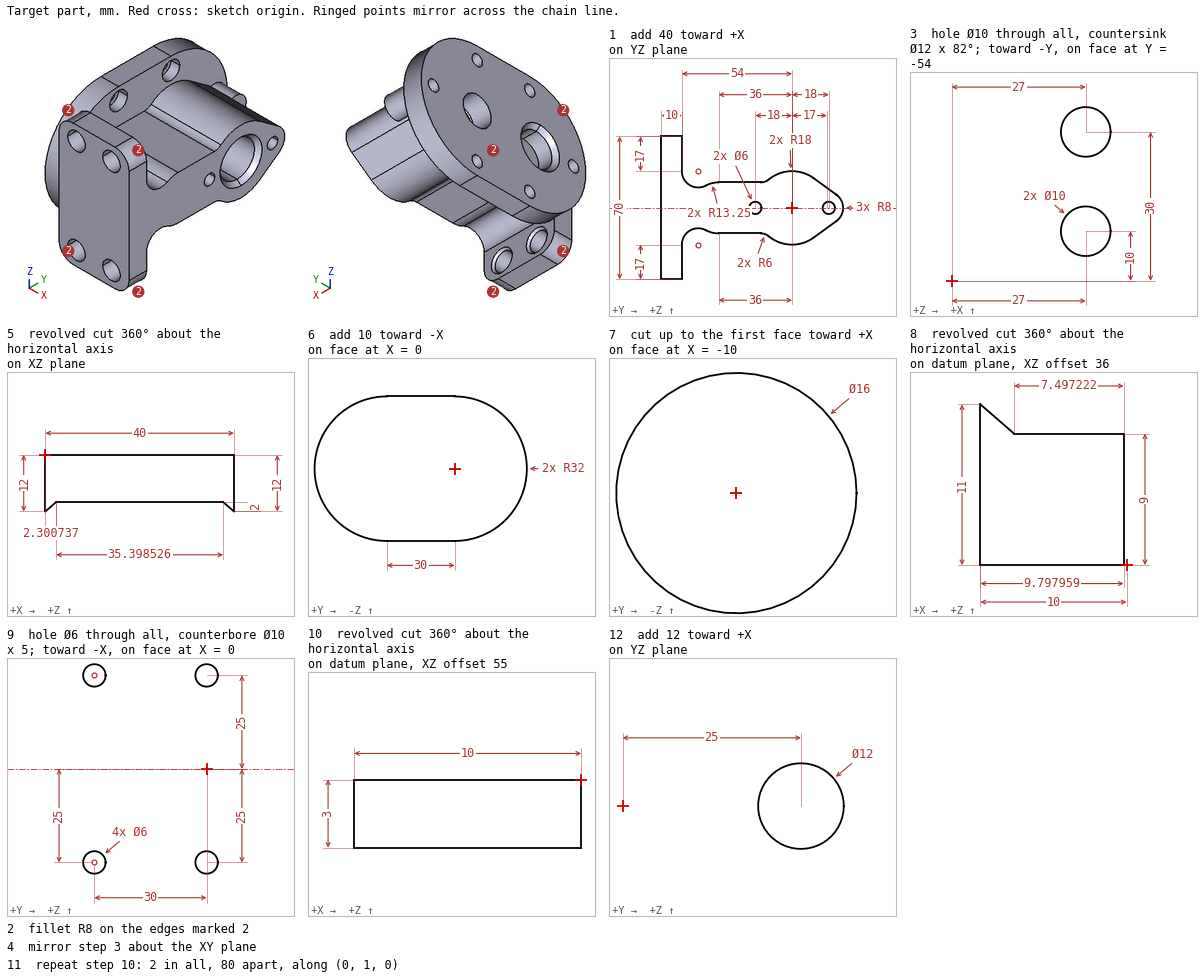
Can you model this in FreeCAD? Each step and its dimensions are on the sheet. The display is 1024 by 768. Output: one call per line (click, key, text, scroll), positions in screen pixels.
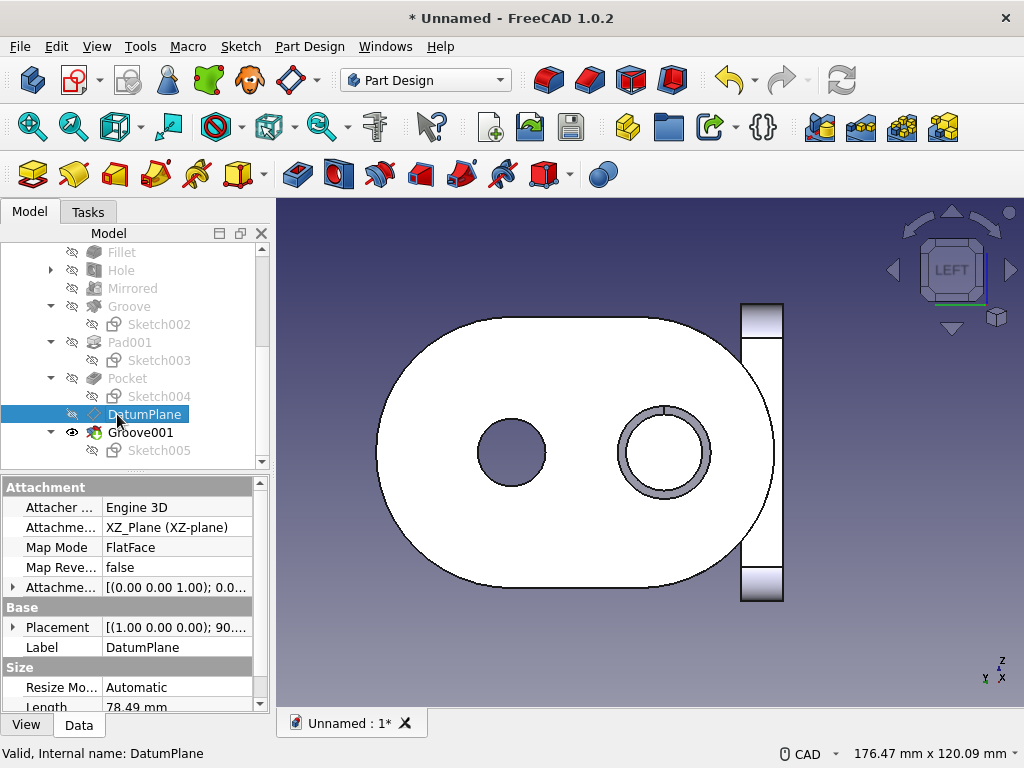
key(0)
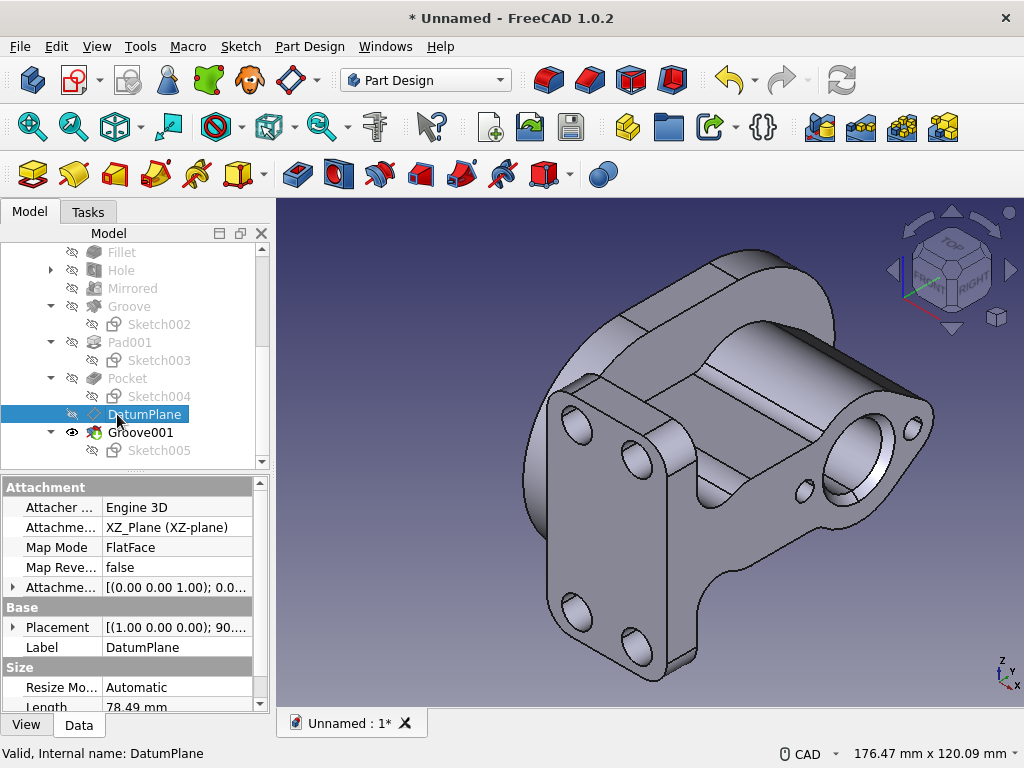
click(33, 128)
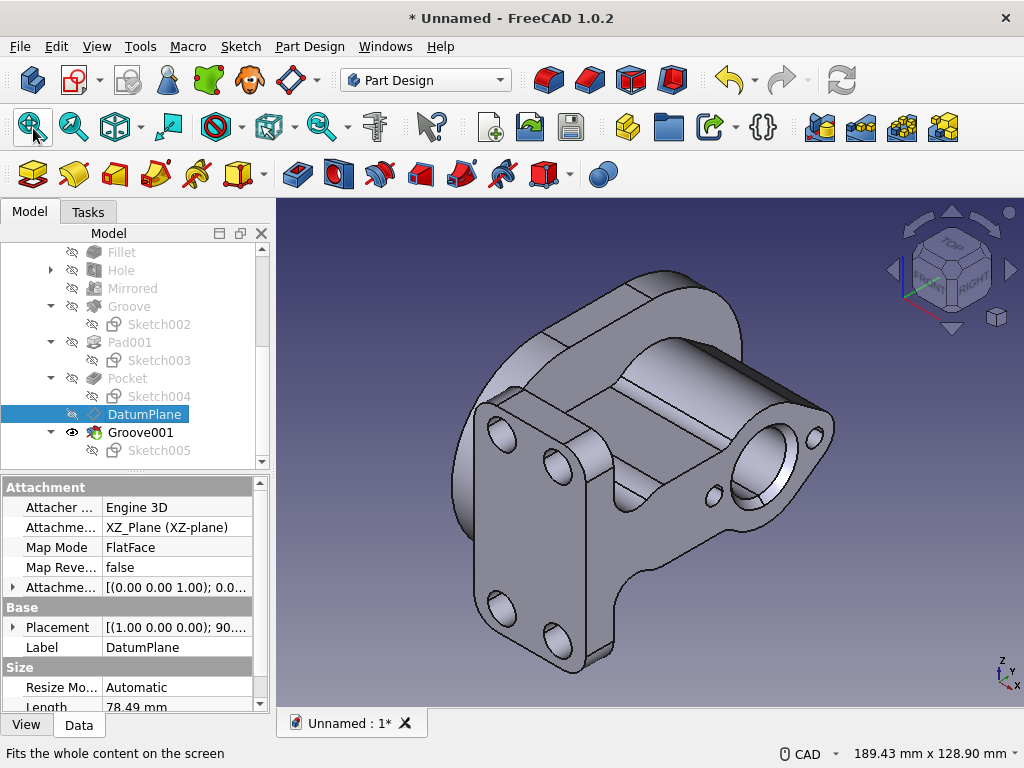
click(588, 380)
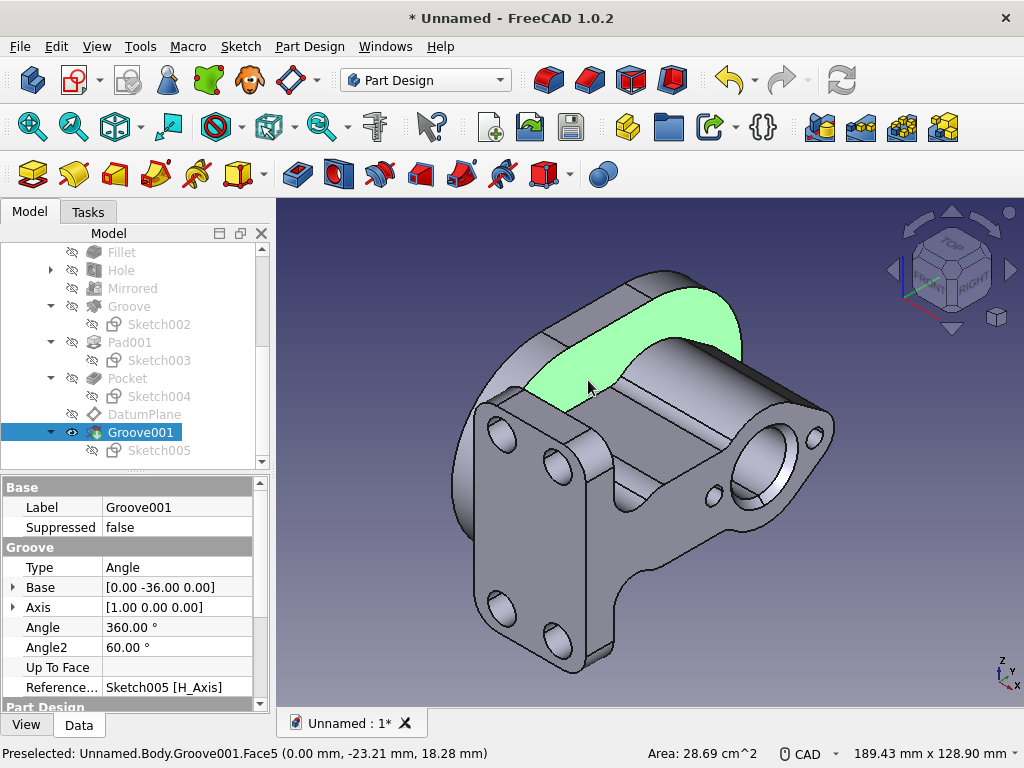
click(74, 80)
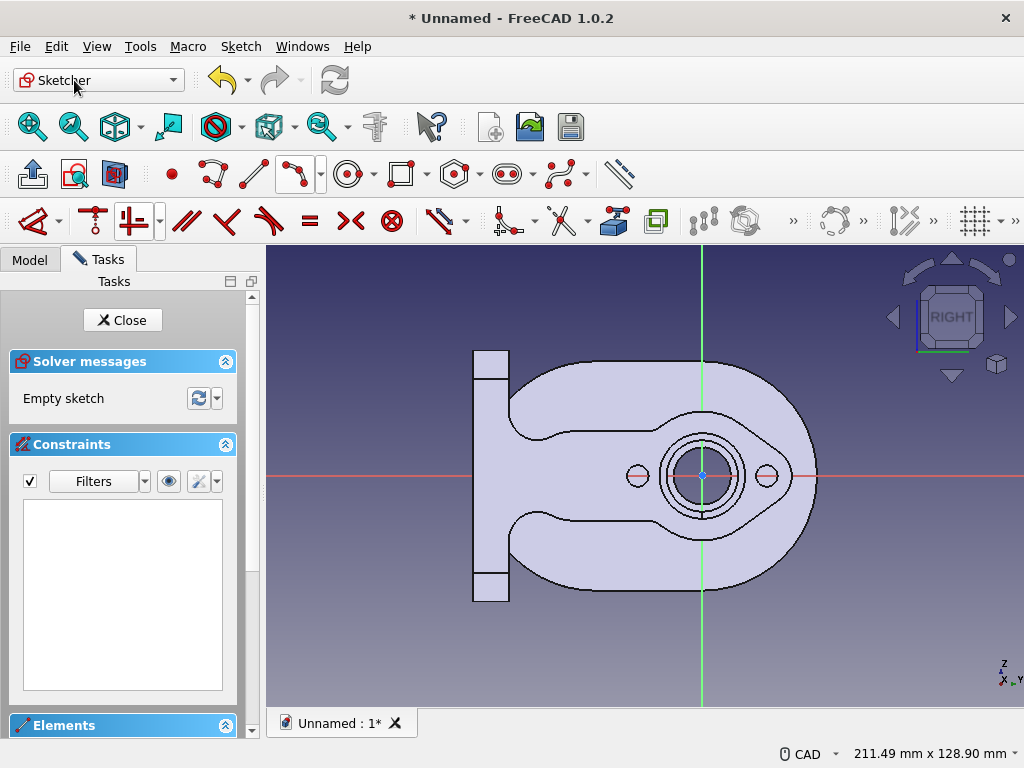
click(115, 174)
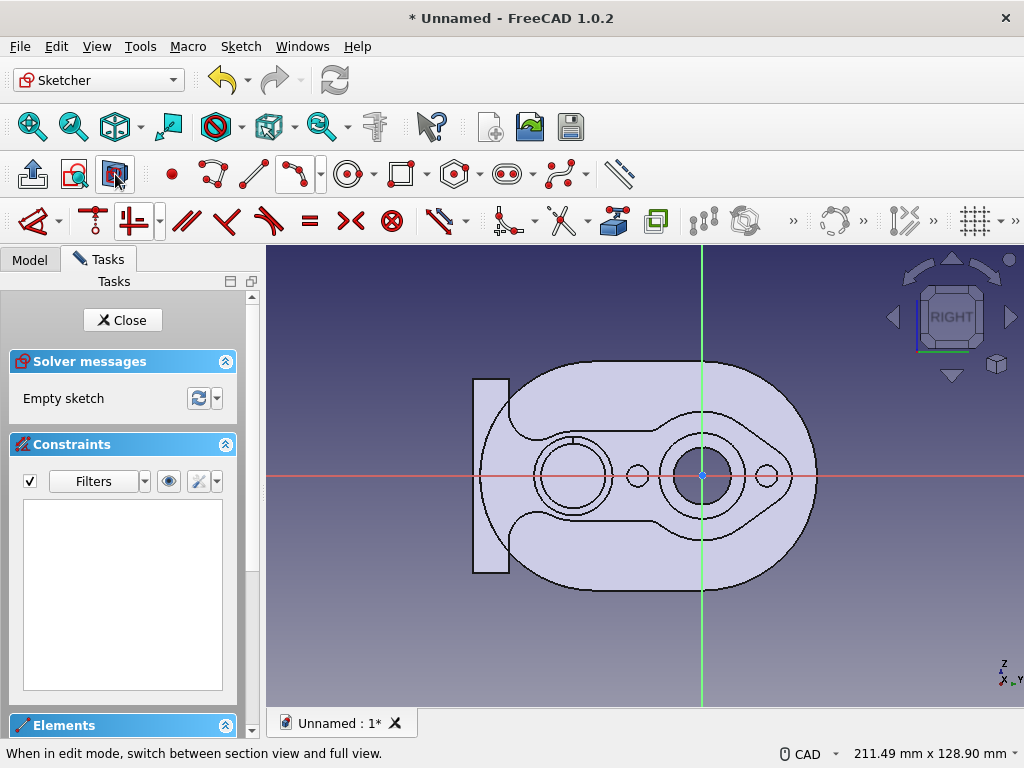
scroll(795, 476, up, 2)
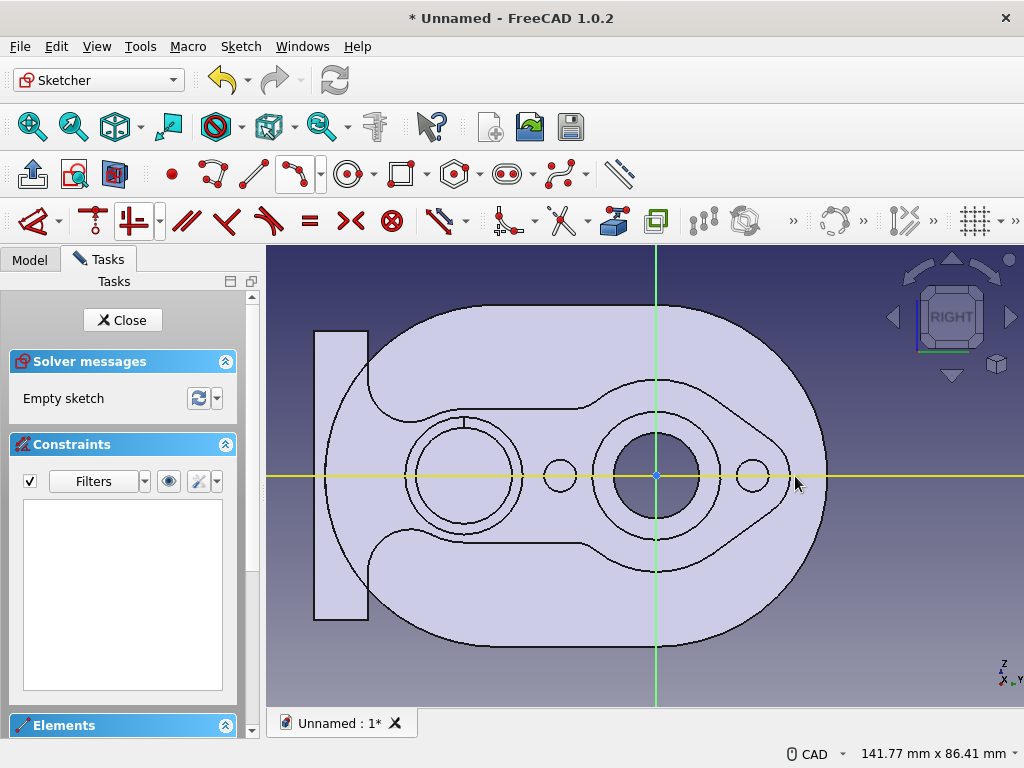
click(348, 174)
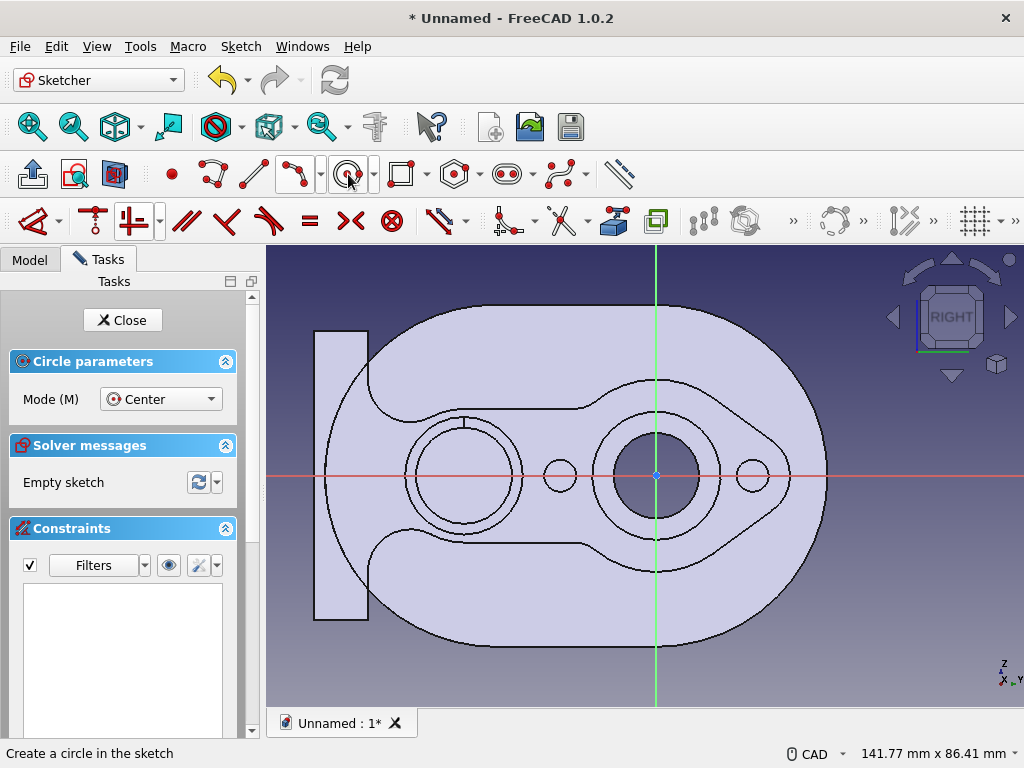
scroll(496, 609, up, 2)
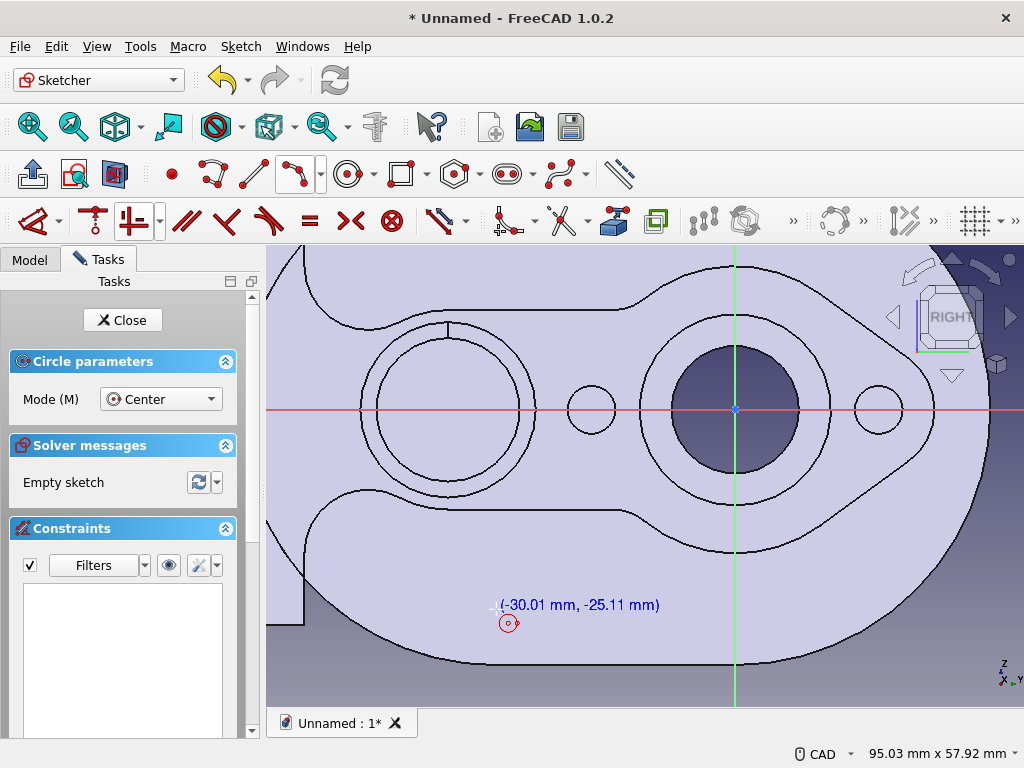
click(496, 609)
click(513, 592)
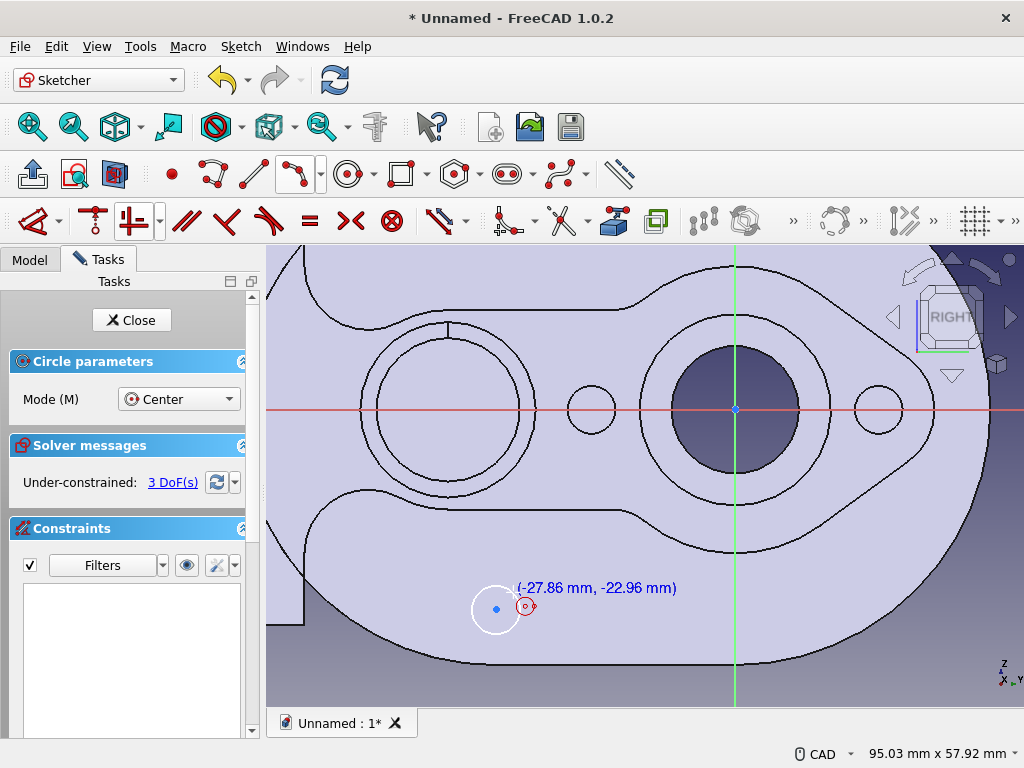
click(735, 609)
click(752, 592)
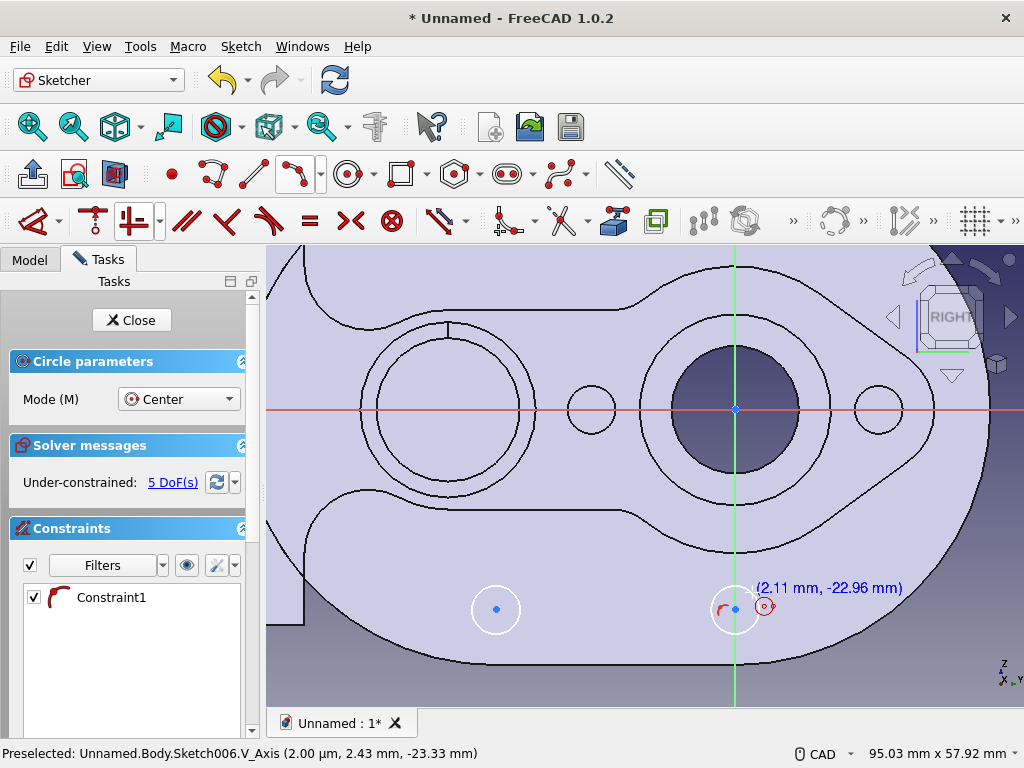
scroll(497, 611, down, 2)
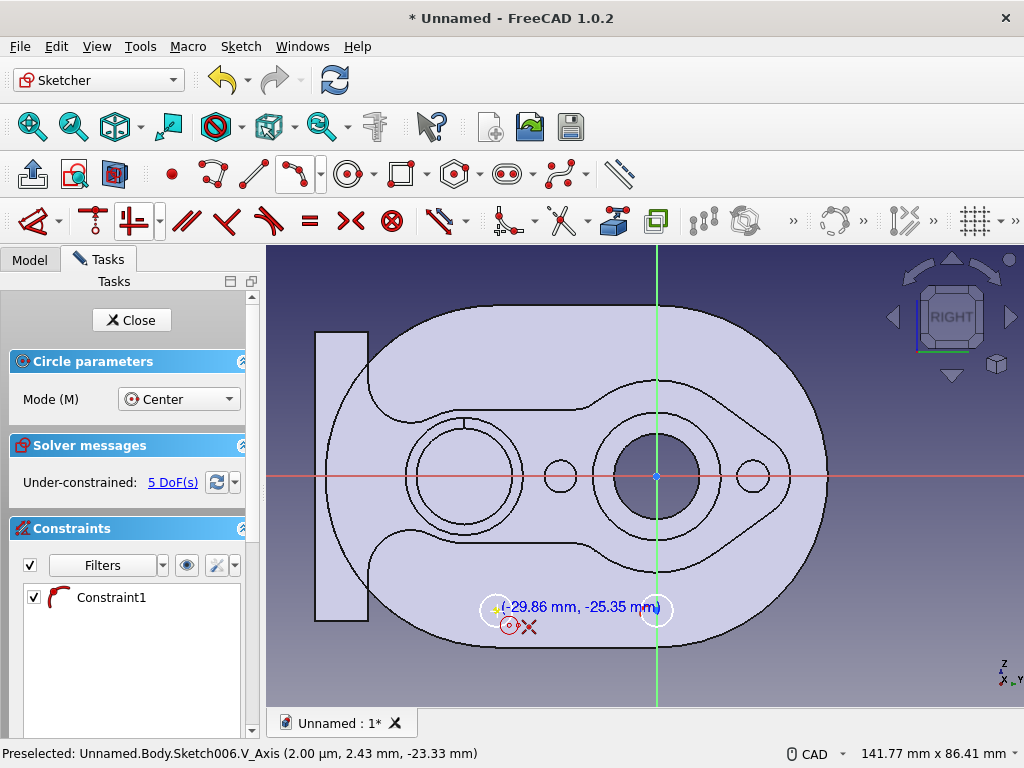
scroll(496, 343, up, 2)